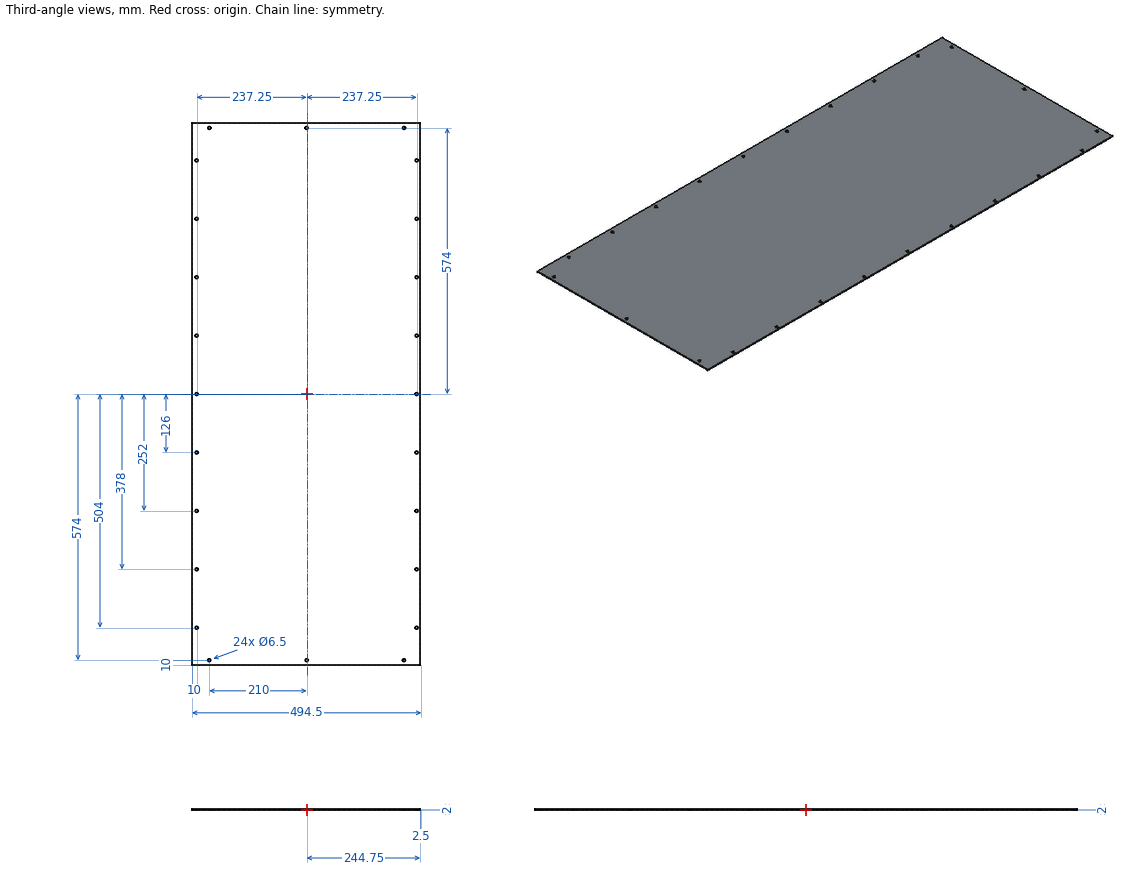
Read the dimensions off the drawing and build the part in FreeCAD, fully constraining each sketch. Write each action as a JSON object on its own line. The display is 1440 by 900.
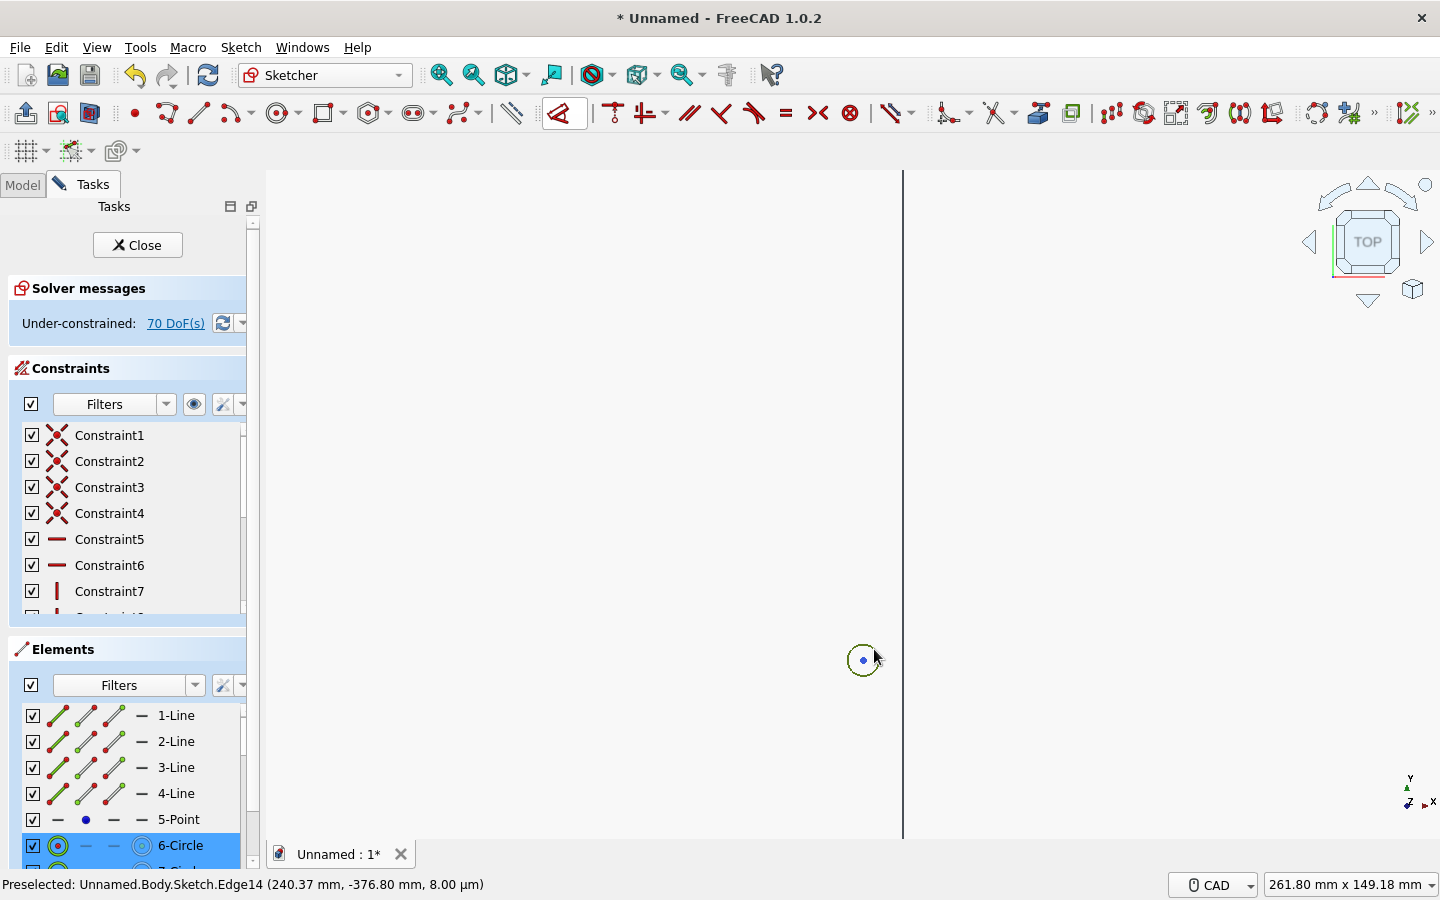
{"action": "scroll", "coordinate": [883, 658], "scroll_direction": "down", "scroll_amount": 12}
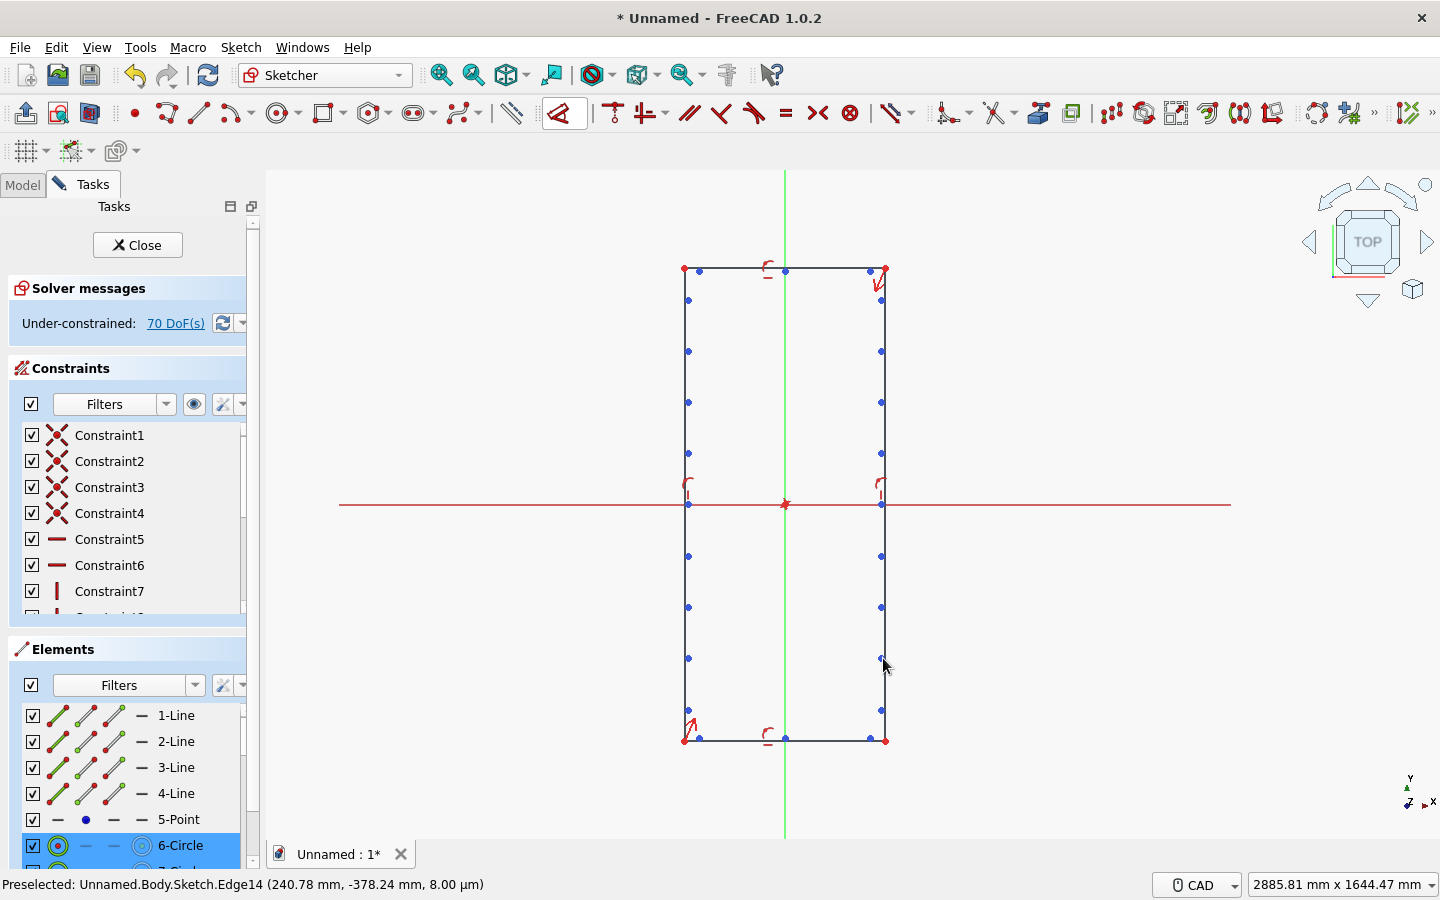
{"action": "scroll", "coordinate": [883, 607], "scroll_direction": "up", "scroll_amount": 11}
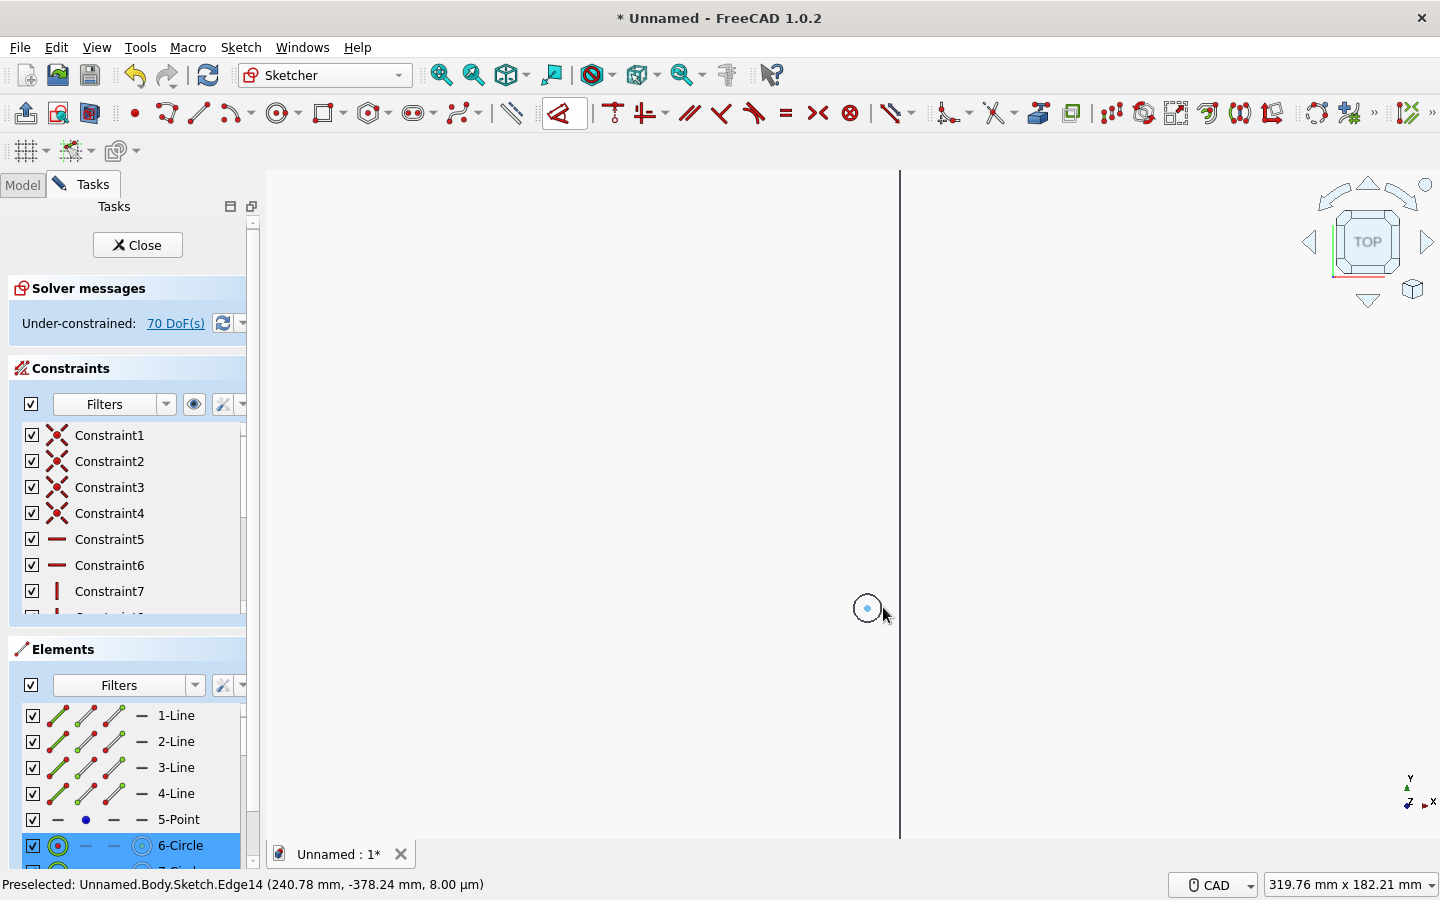
{"action": "left_click", "coordinate": [877, 598]}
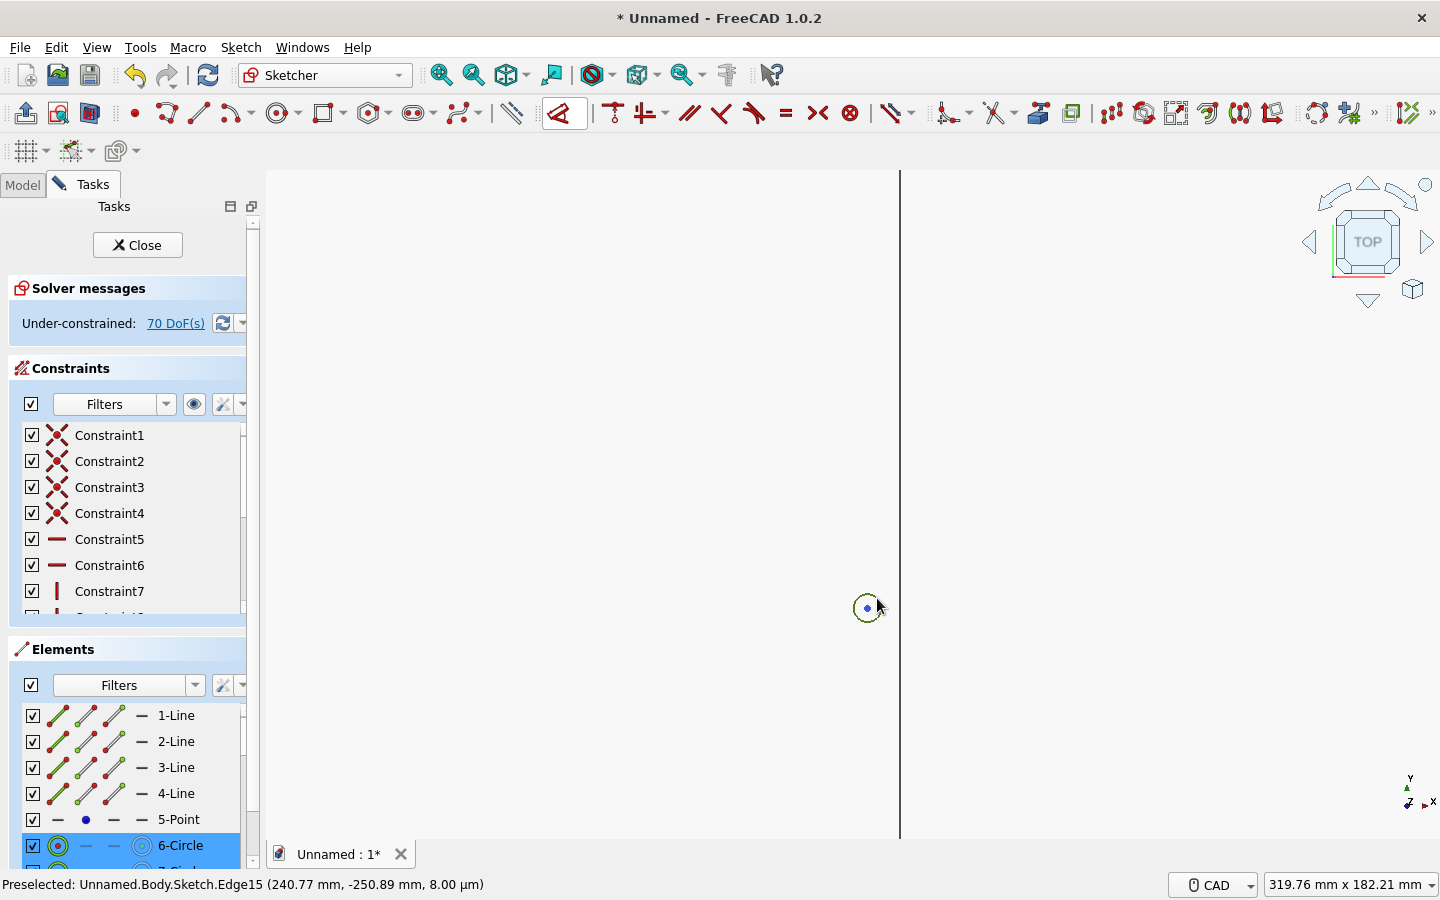
{"action": "scroll", "coordinate": [883, 607], "scroll_direction": "down", "scroll_amount": 11}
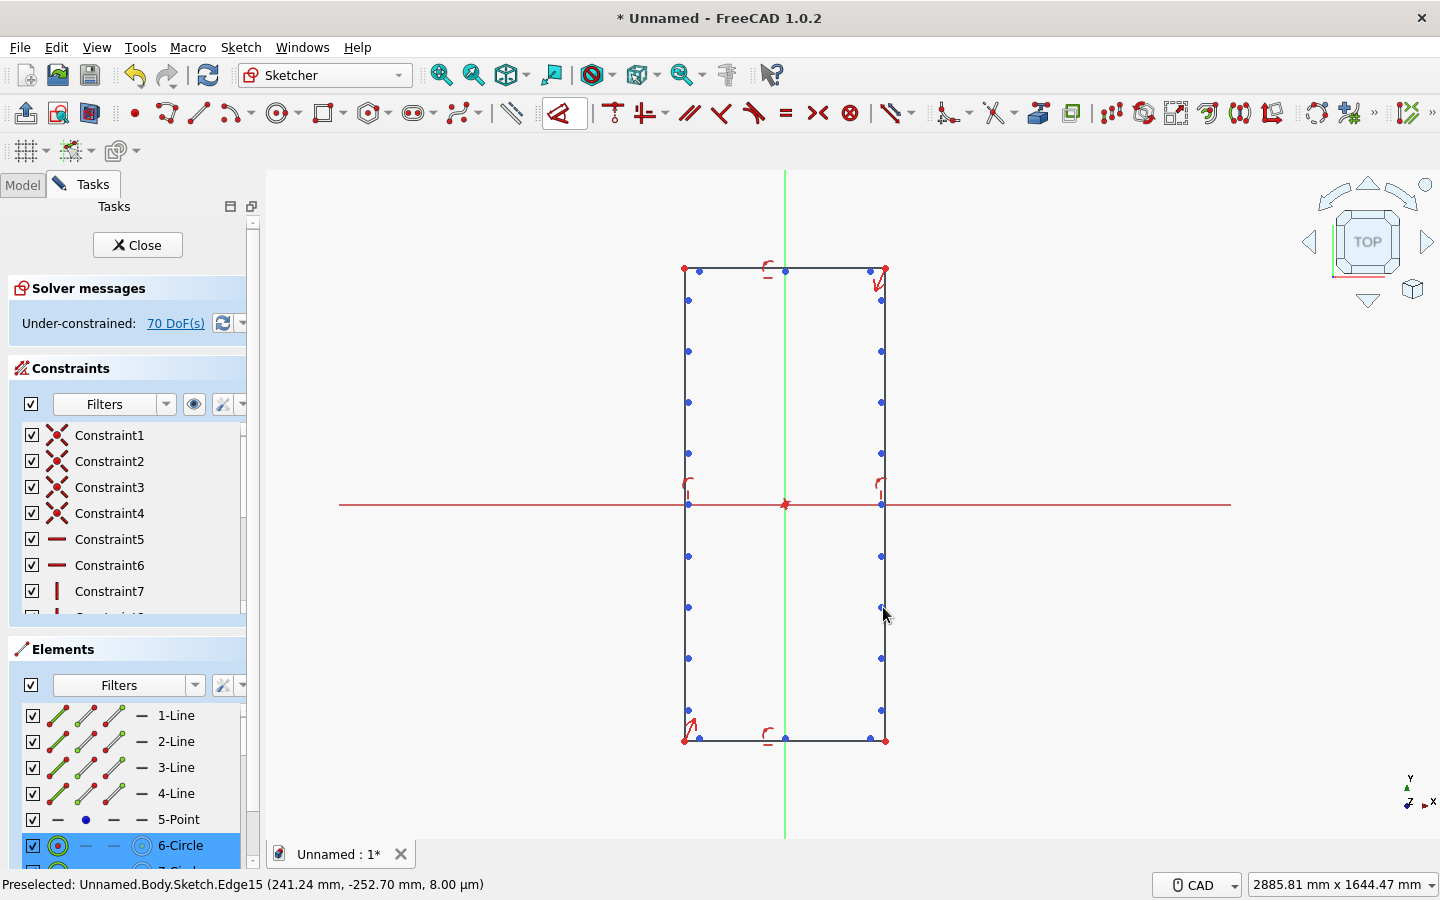
{"action": "scroll", "coordinate": [883, 555], "scroll_direction": "up", "scroll_amount": 12}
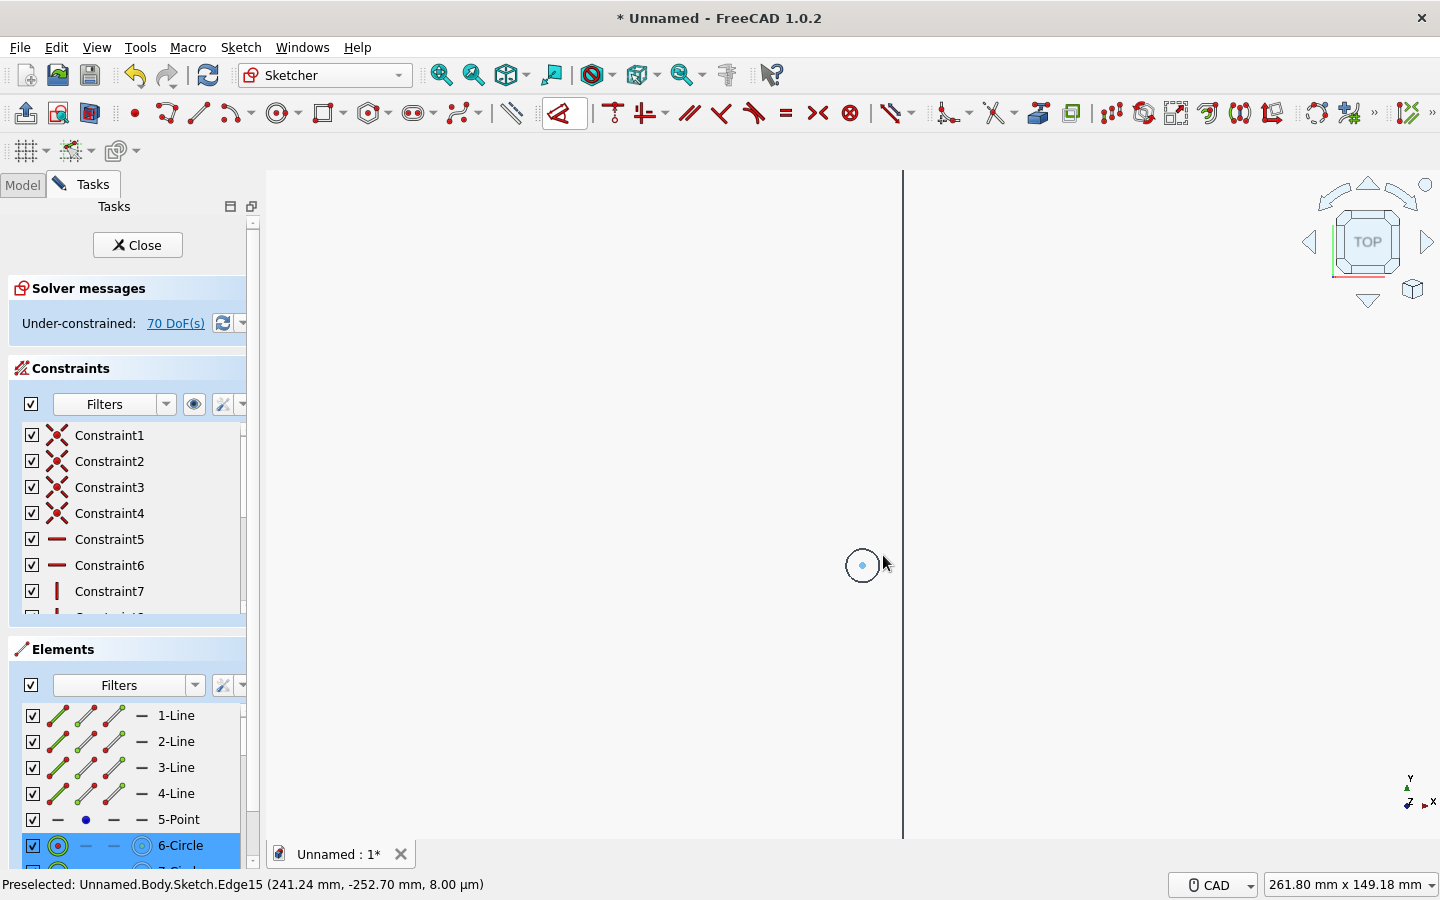
{"action": "left_click", "coordinate": [874, 554]}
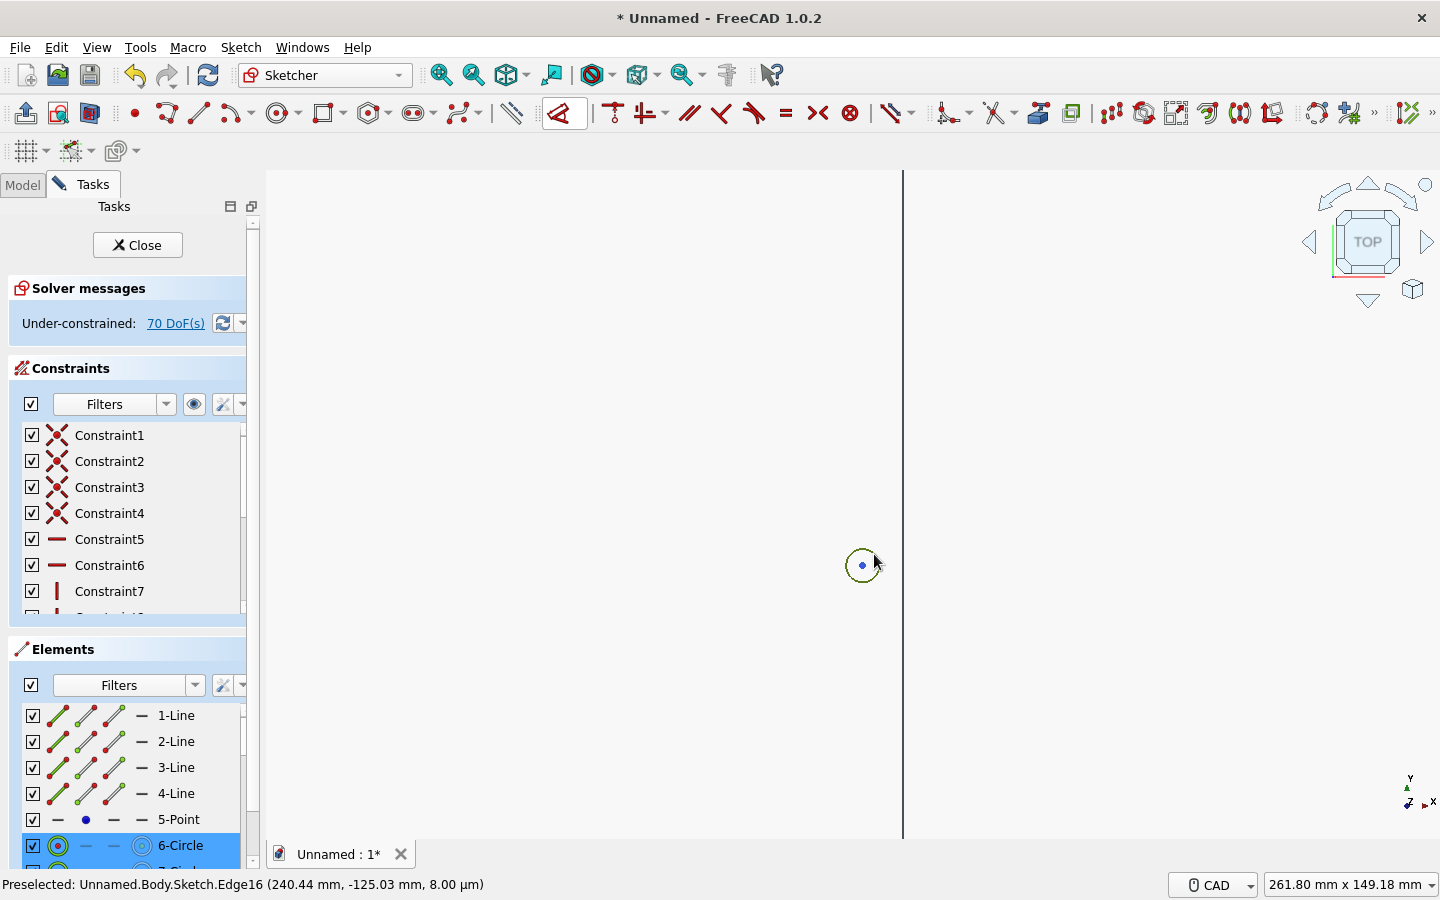
{"action": "scroll", "coordinate": [883, 555], "scroll_direction": "down", "scroll_amount": 12}